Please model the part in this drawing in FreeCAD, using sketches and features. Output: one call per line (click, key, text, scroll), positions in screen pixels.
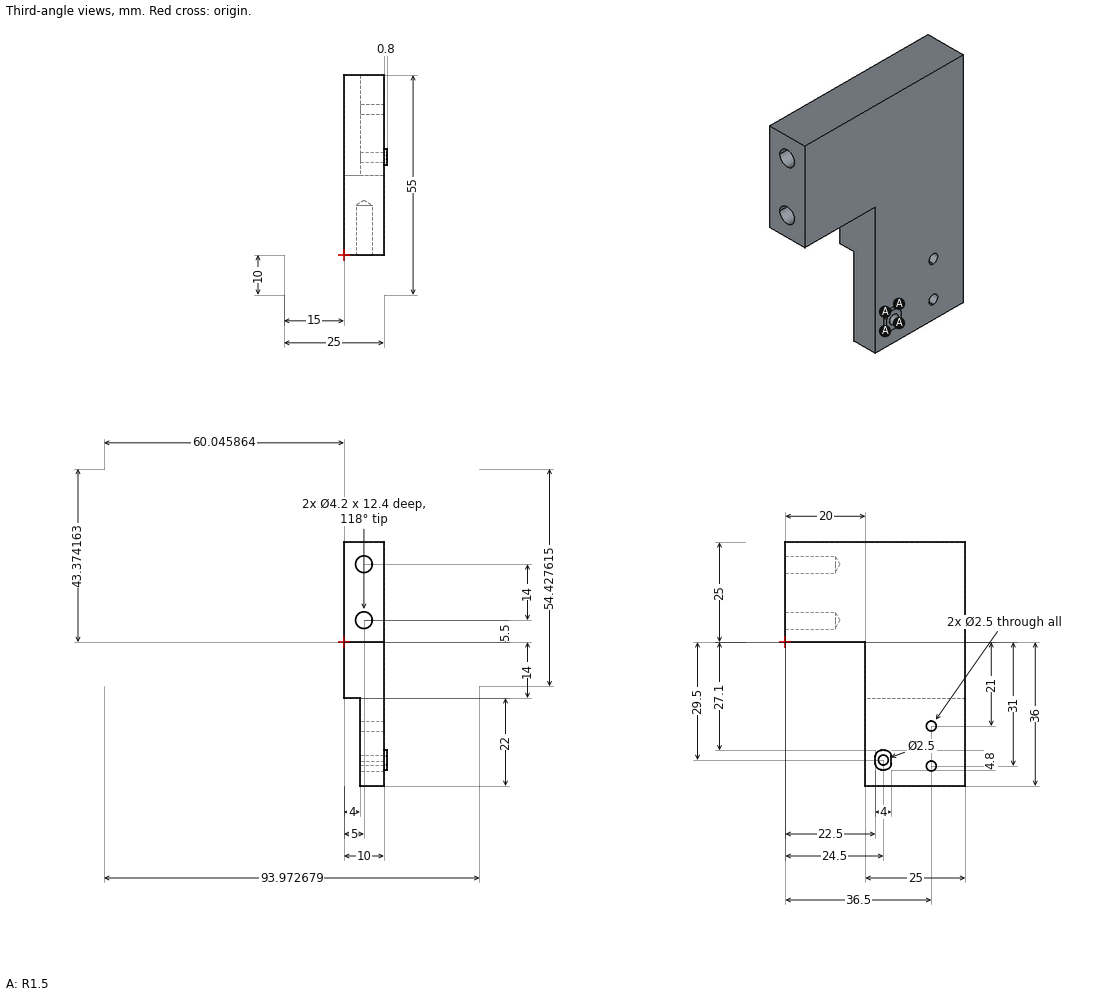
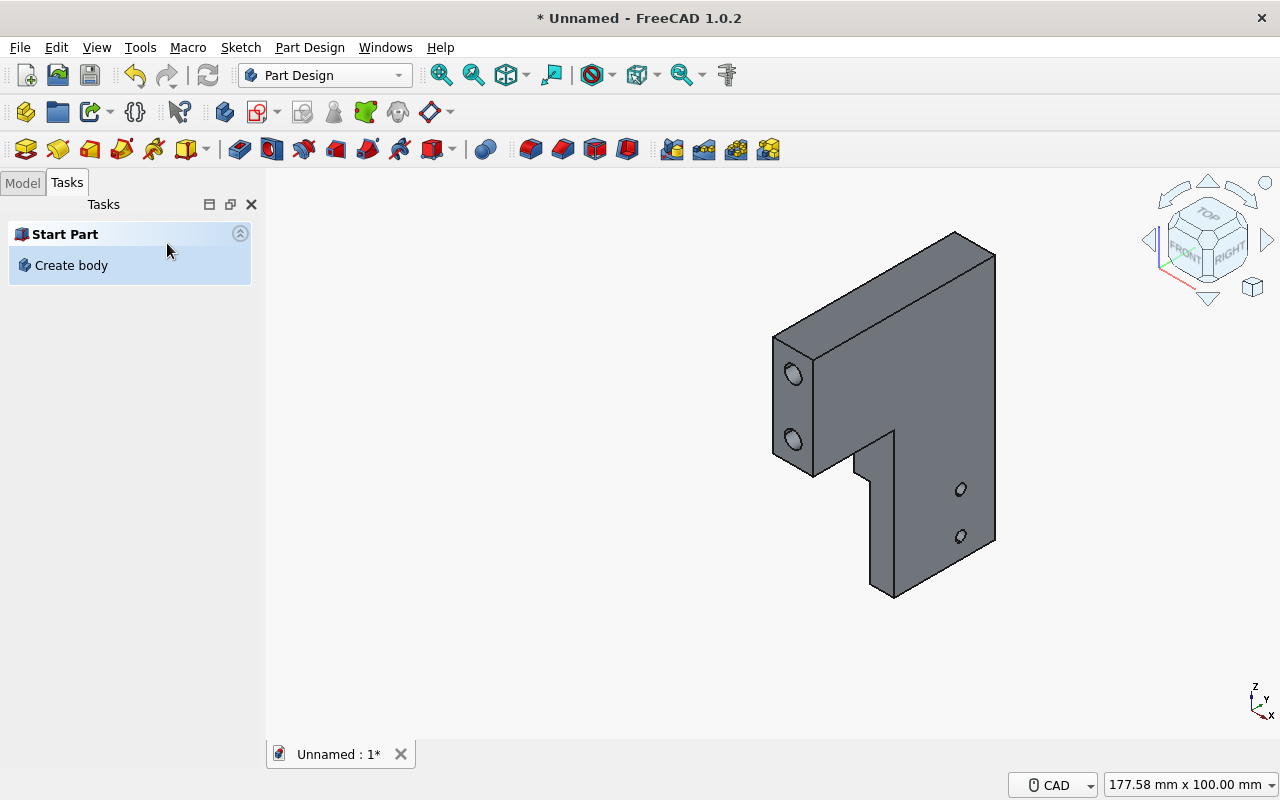
click(930, 353)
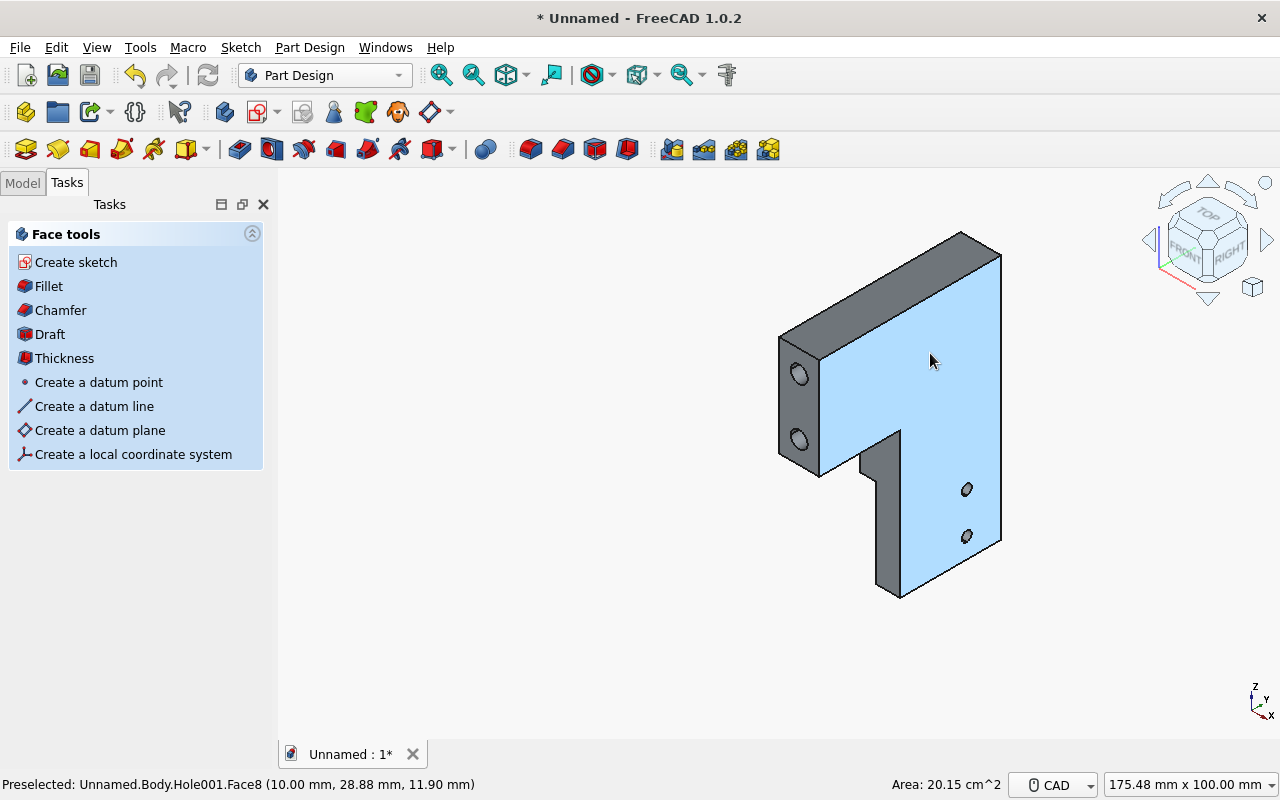
click(258, 112)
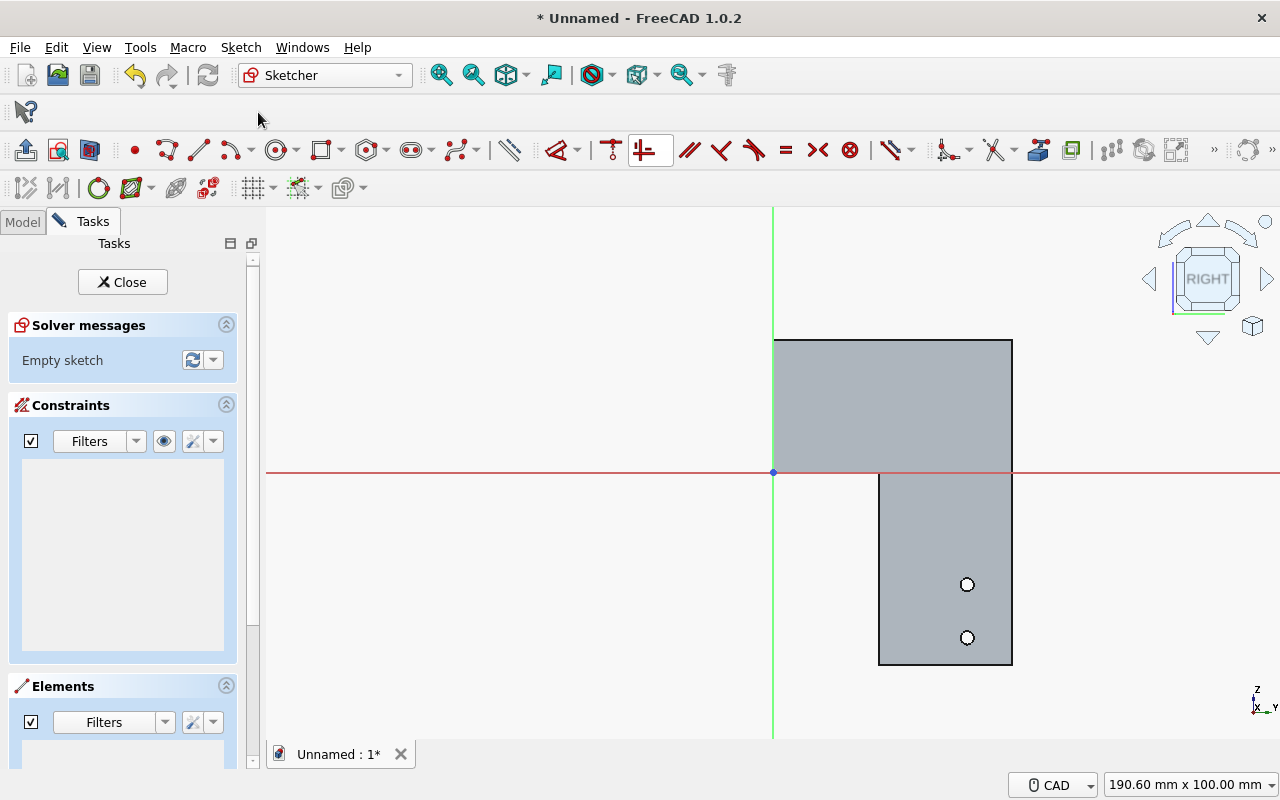
scroll(919, 643, up, 13)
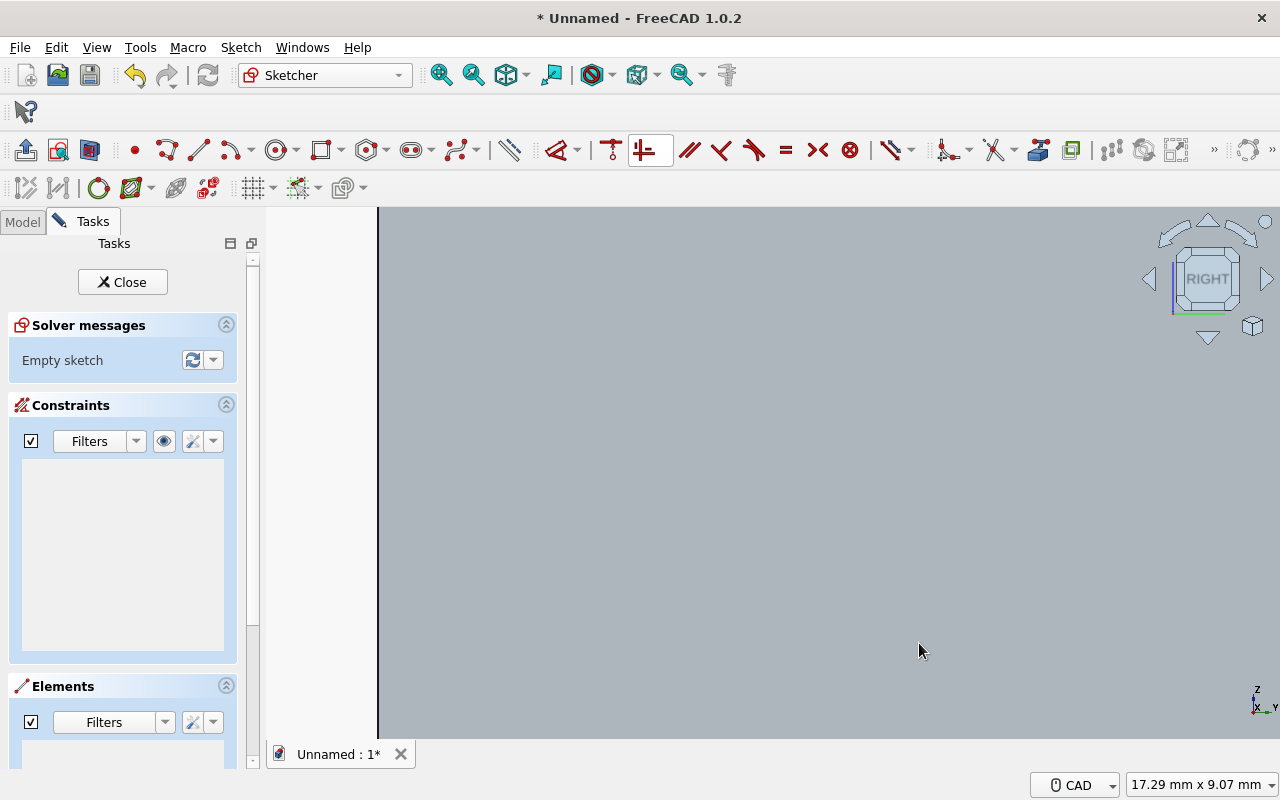
click(322, 150)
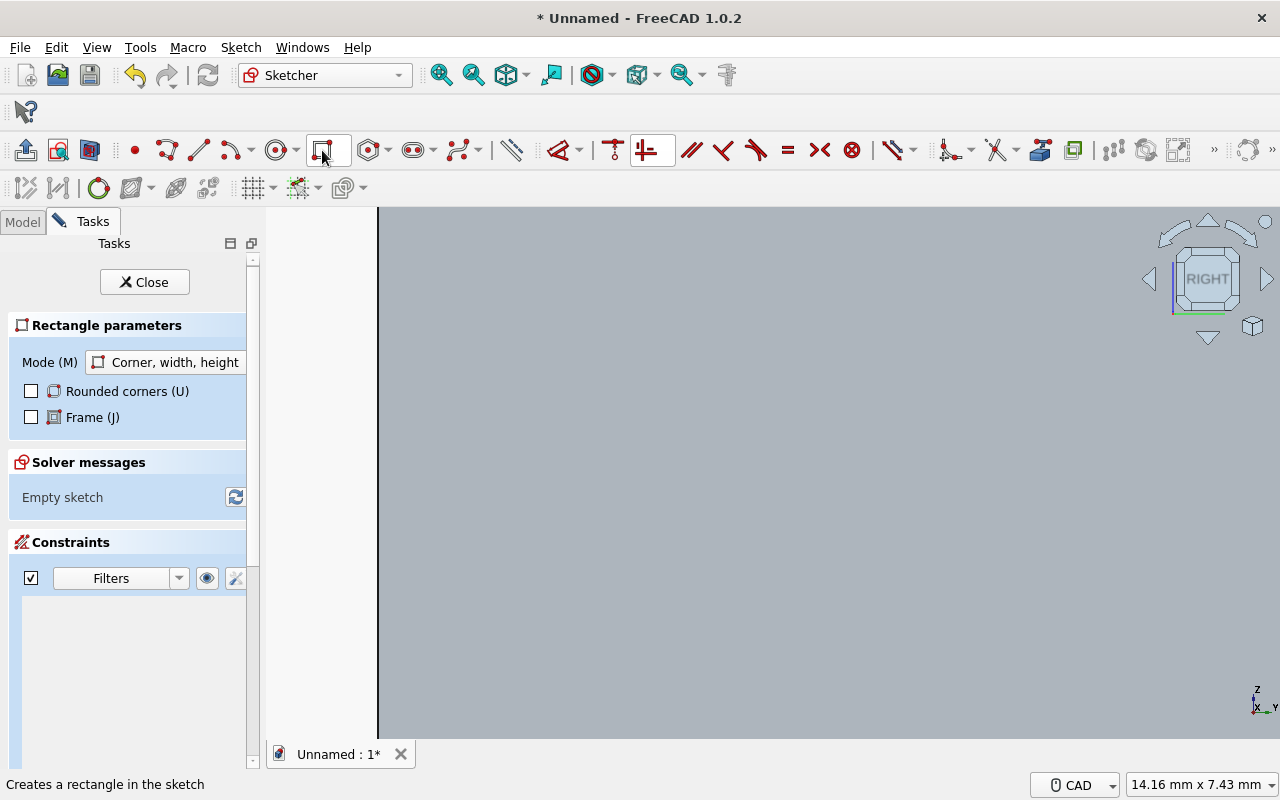
click(557, 285)
move(843, 629)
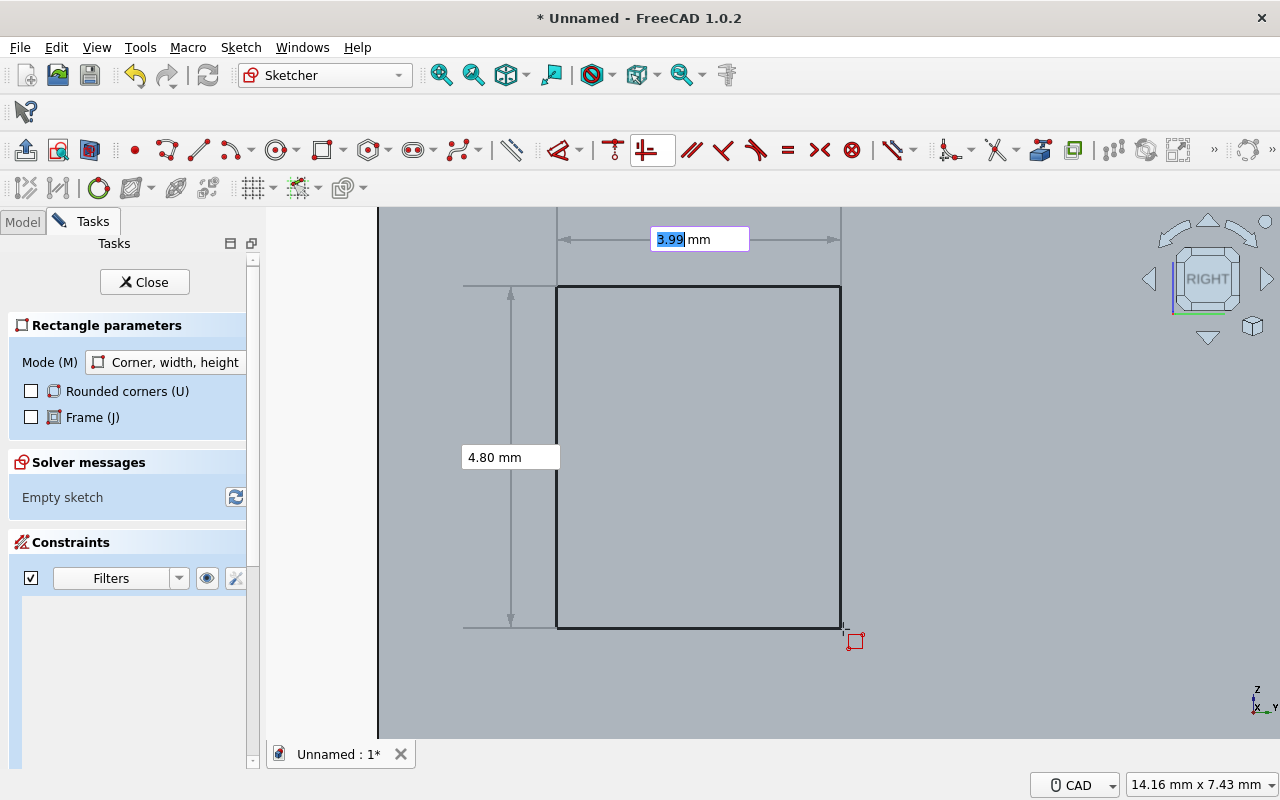
text(4)
key(Tab)
text(4.8)
key(Return)
key(Escape)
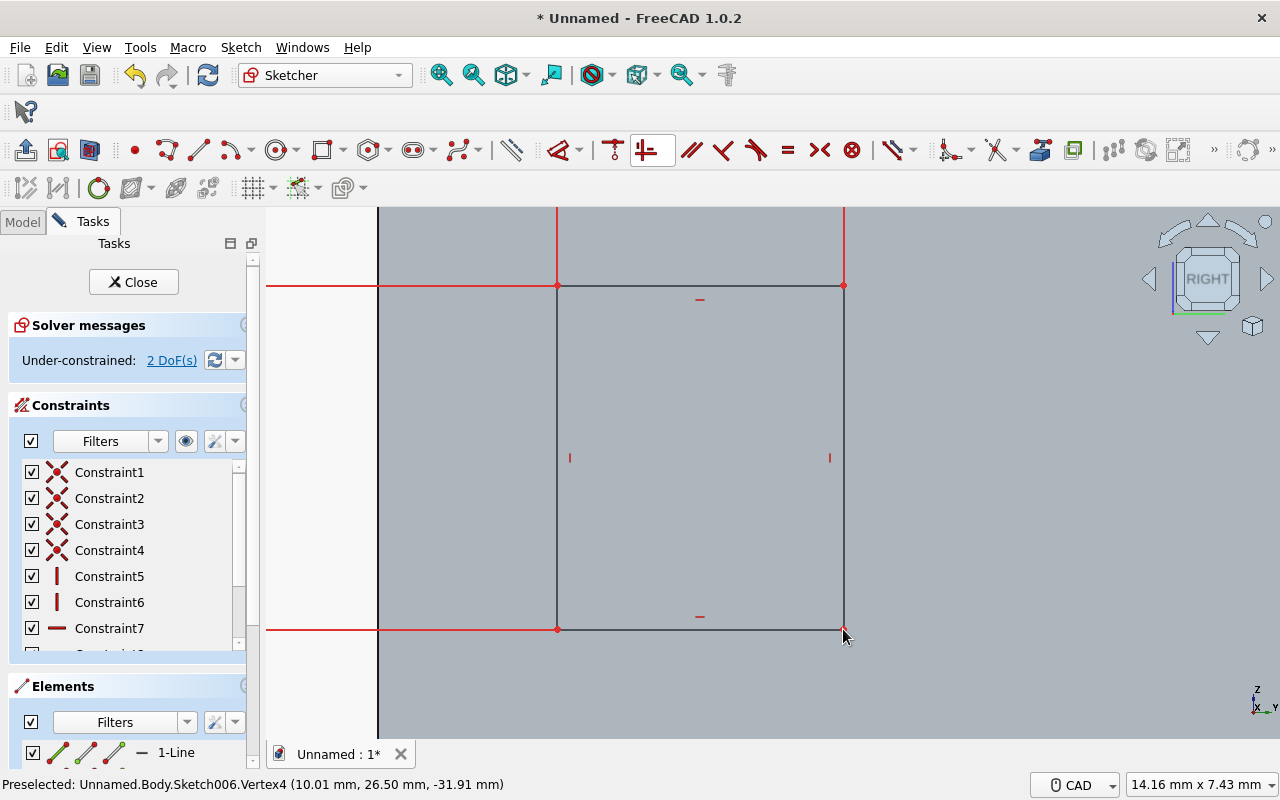
click(558, 150)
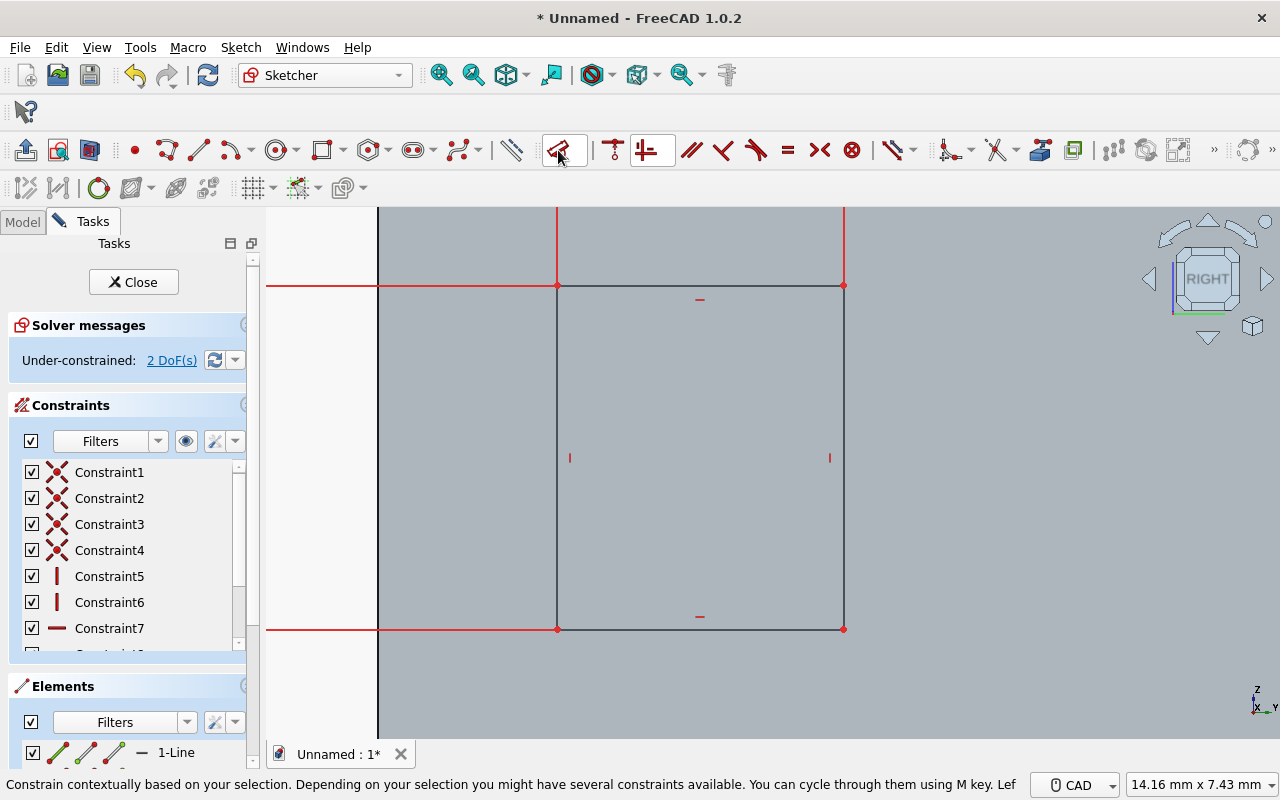
click(557, 286)
click(426, 320)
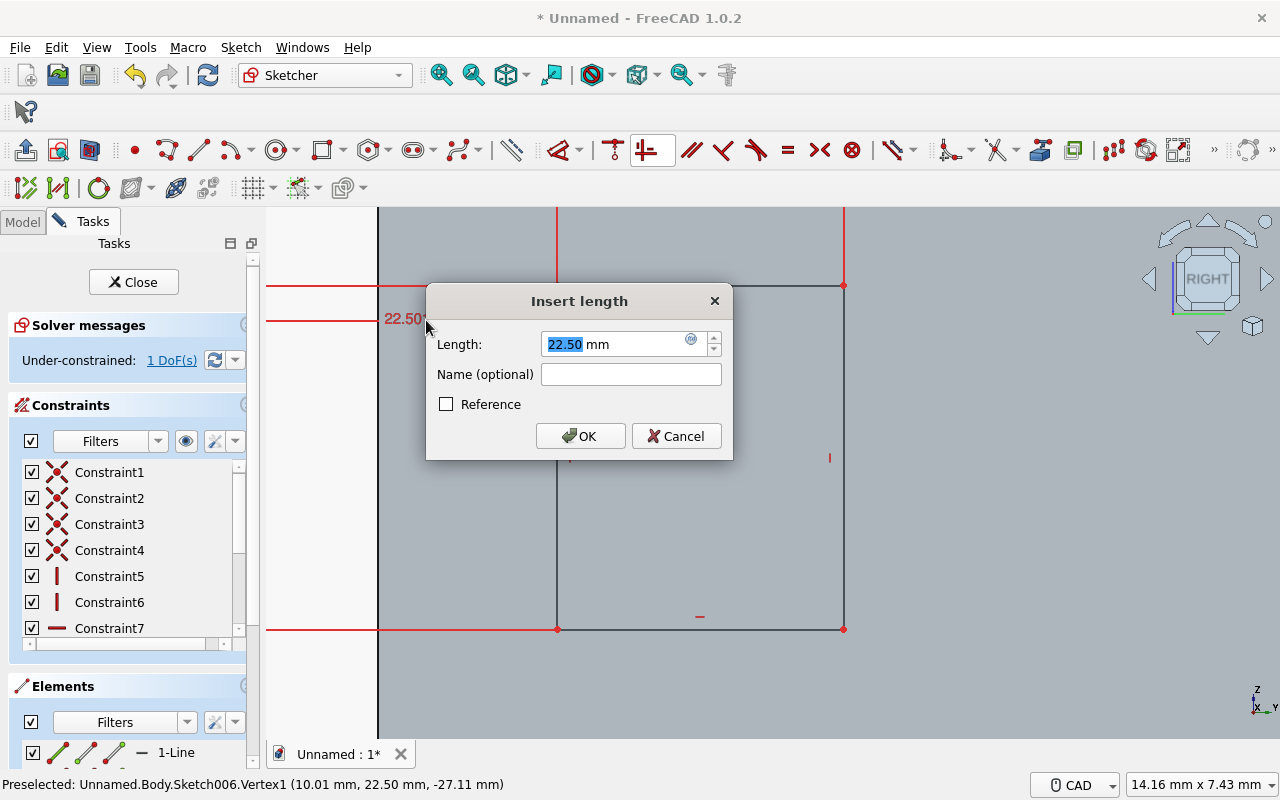
text(22.5)
key(Return)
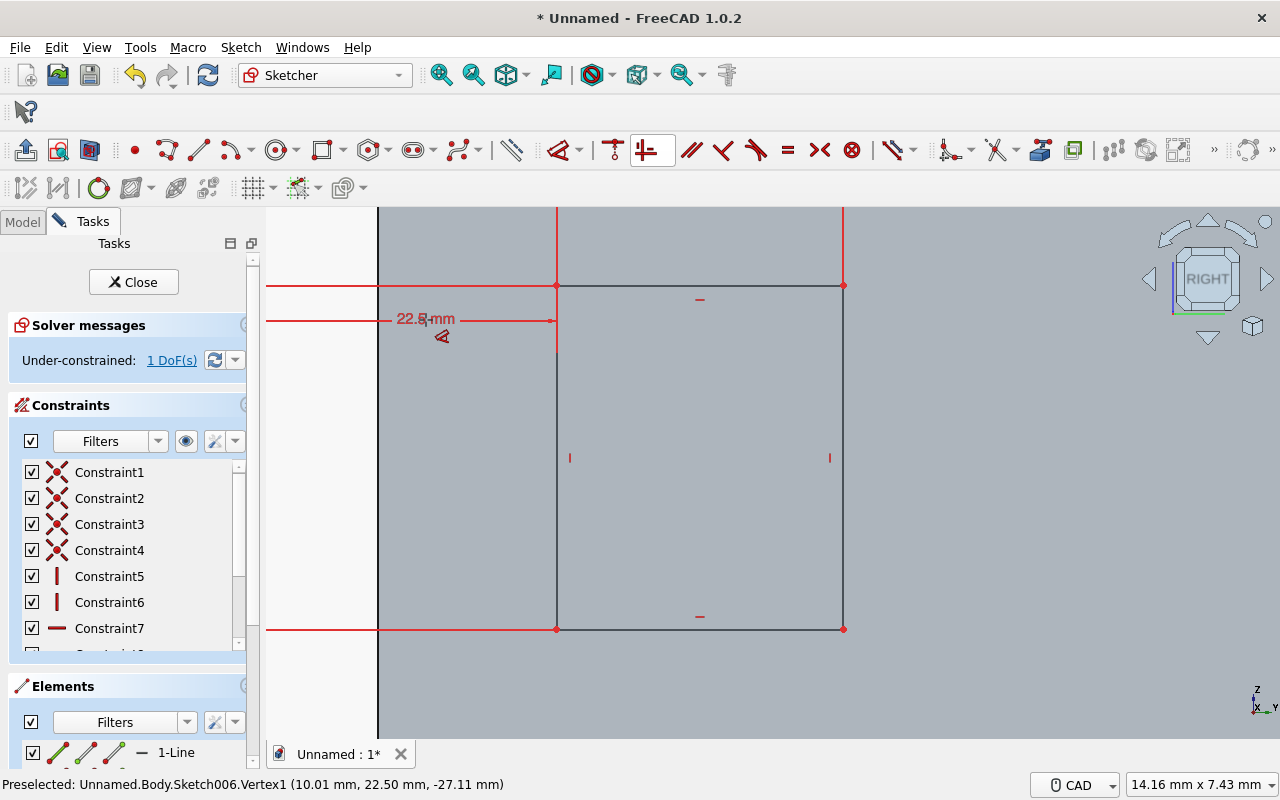
click(557, 286)
click(591, 260)